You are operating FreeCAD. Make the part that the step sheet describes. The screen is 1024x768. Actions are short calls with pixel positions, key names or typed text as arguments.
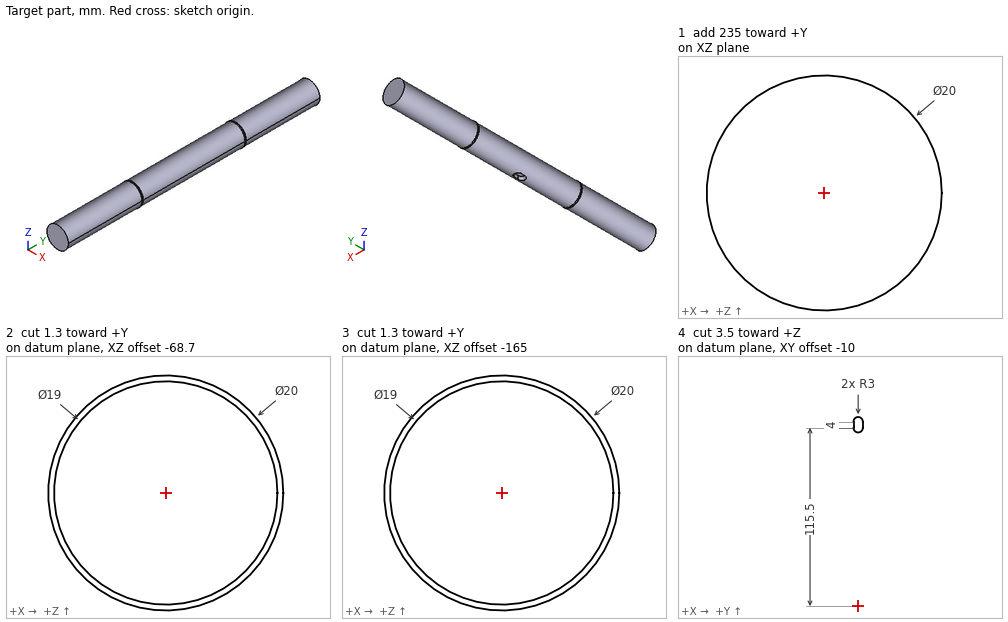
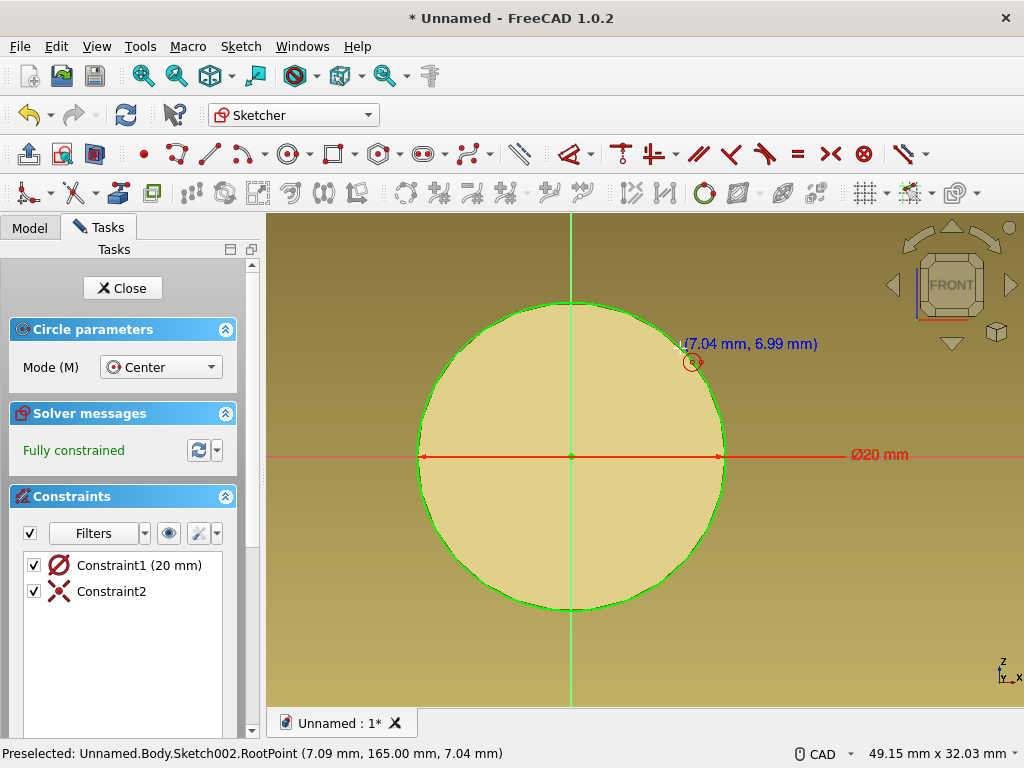
click(571, 457)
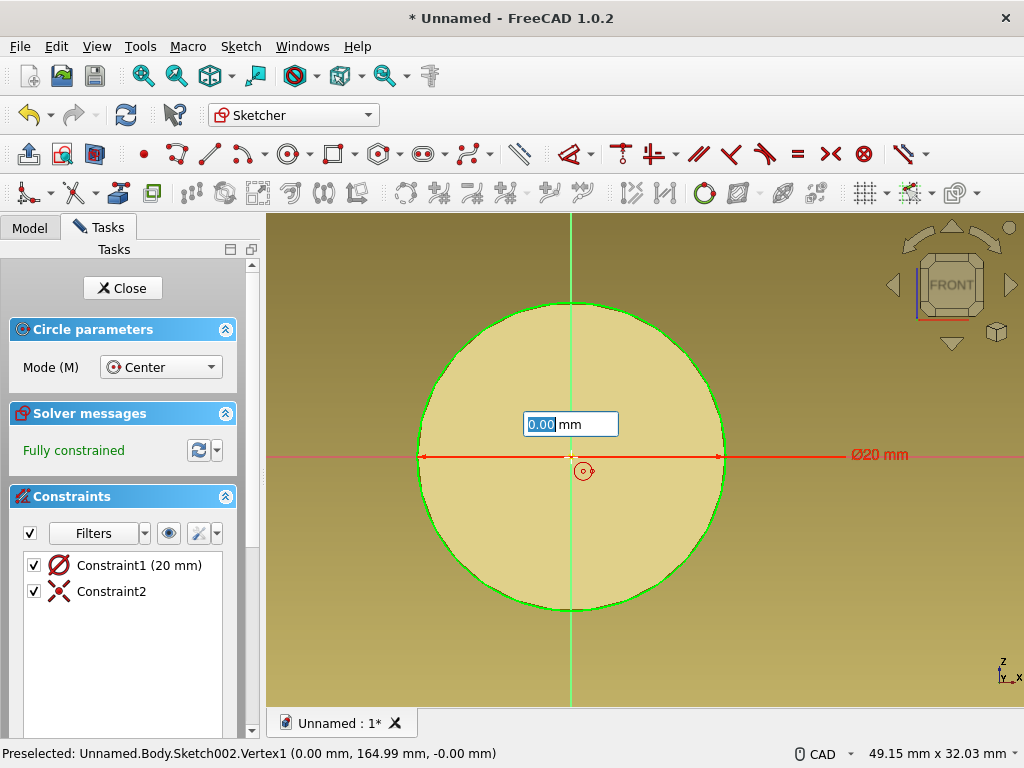
scroll(675, 353, up, 4)
move(674, 353)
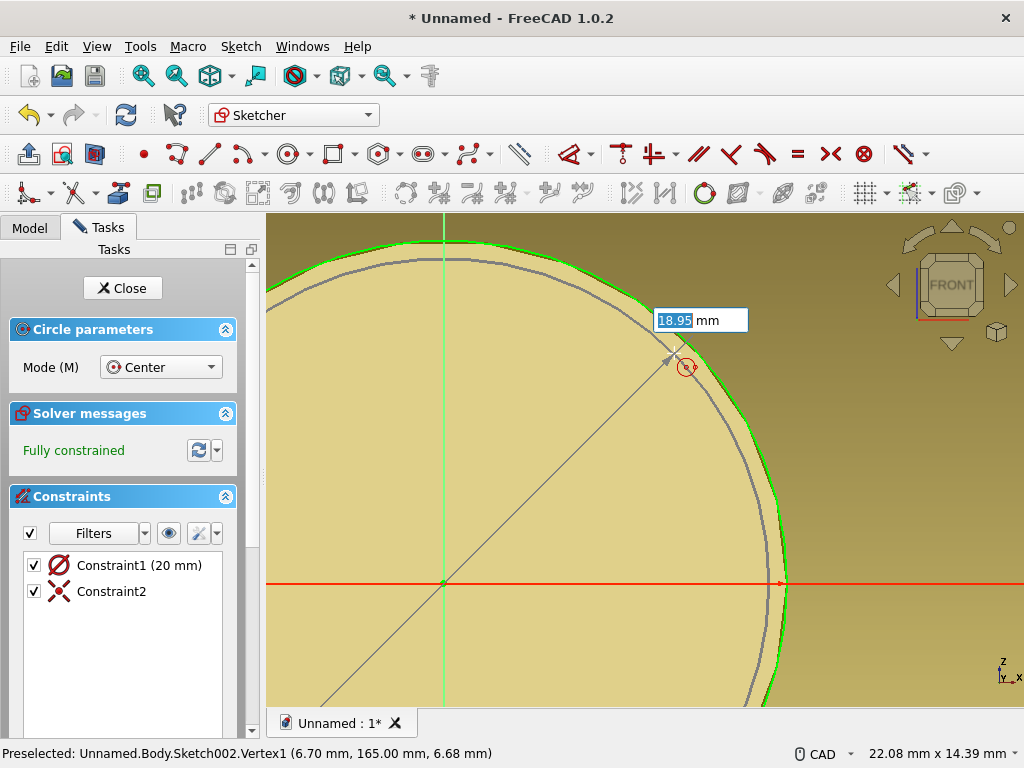
text(19)
key(Return)
key(Escape)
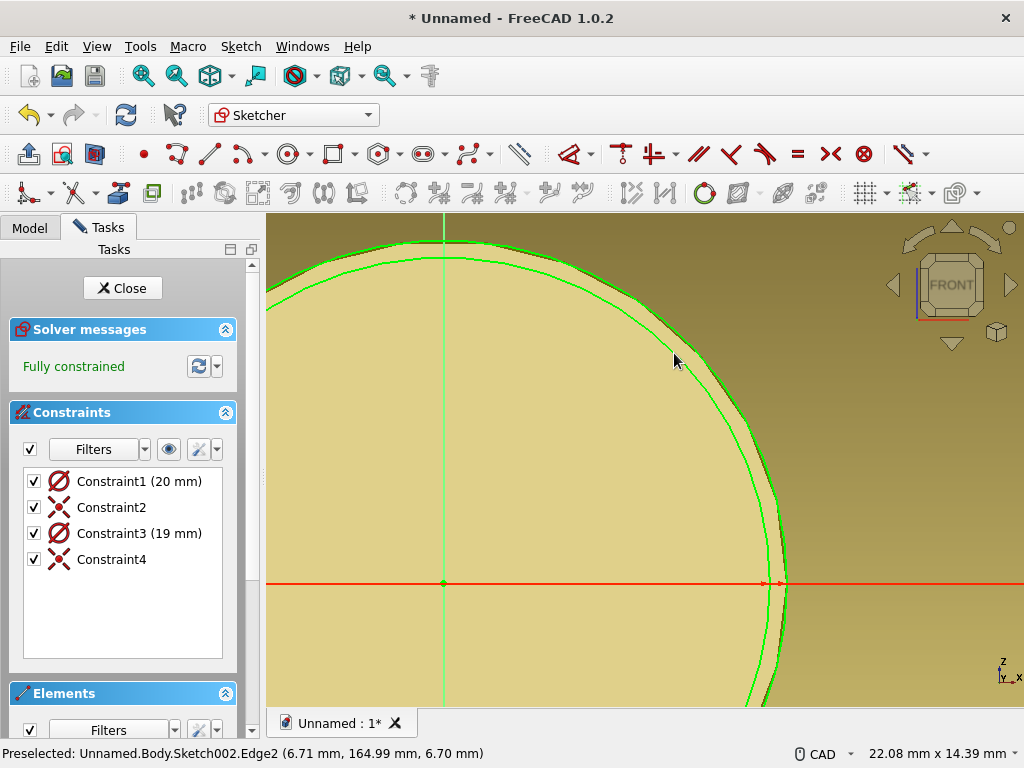
click(123, 288)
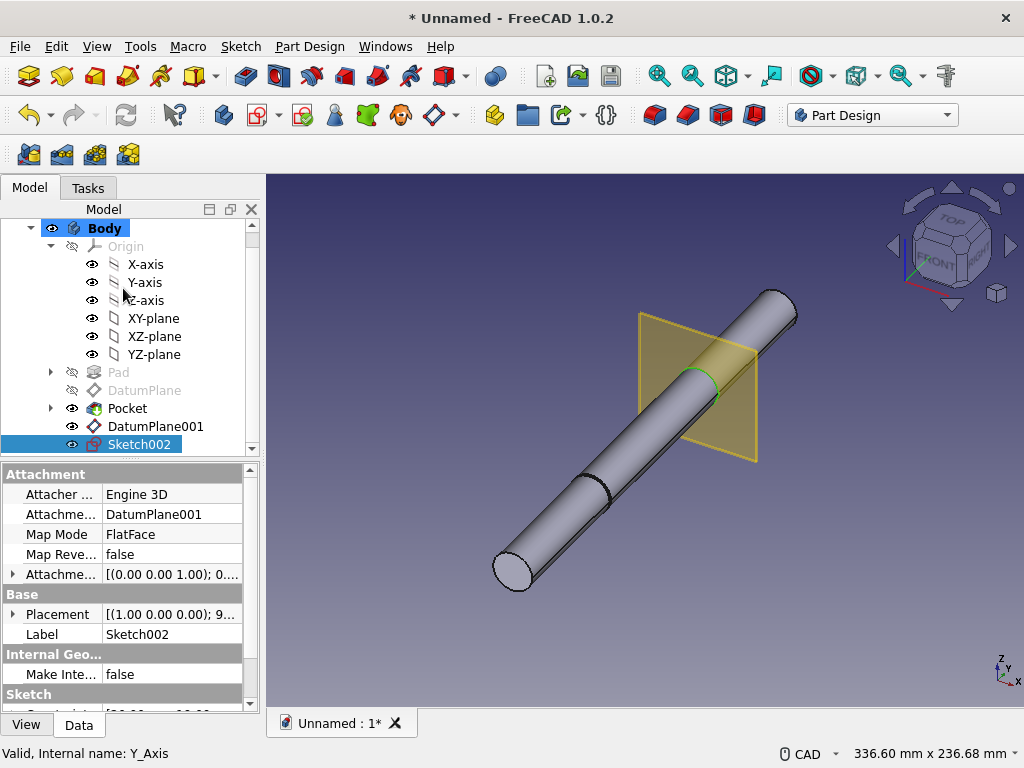
click(246, 76)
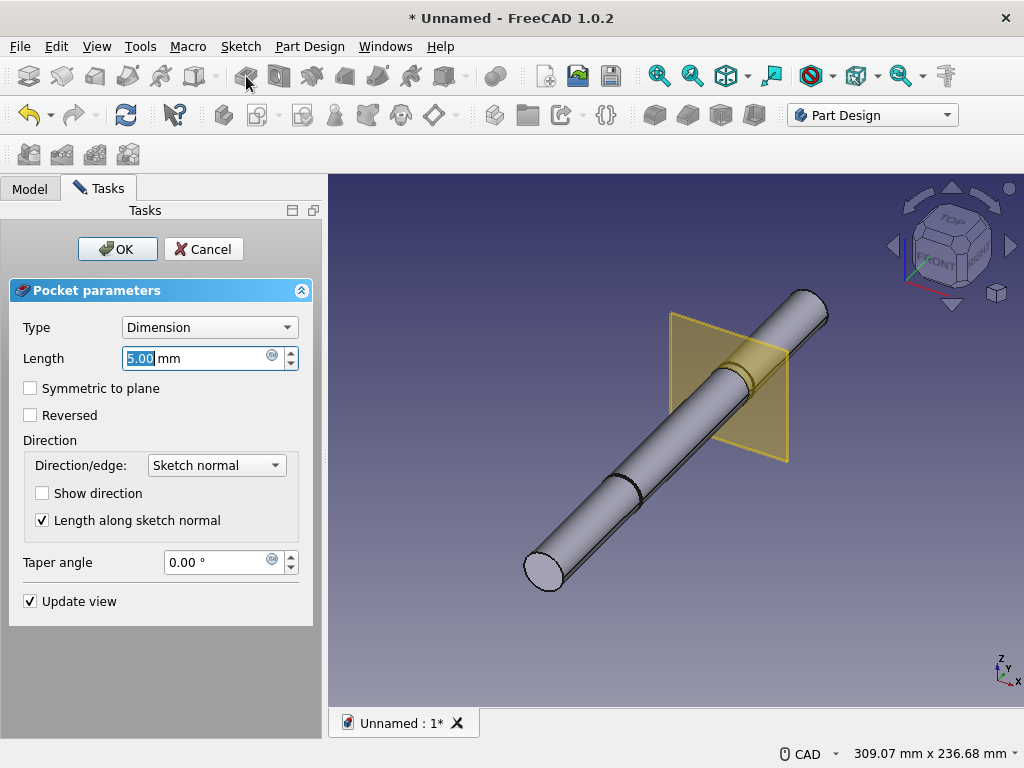
text(1.3)
key(Tab)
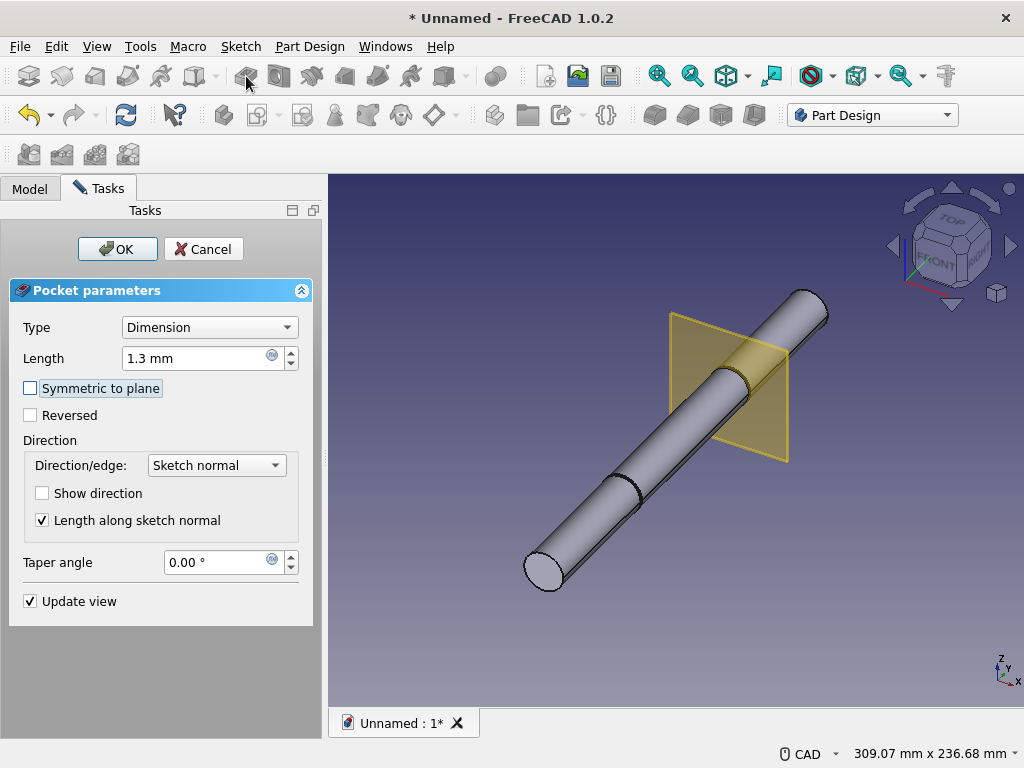
click(118, 249)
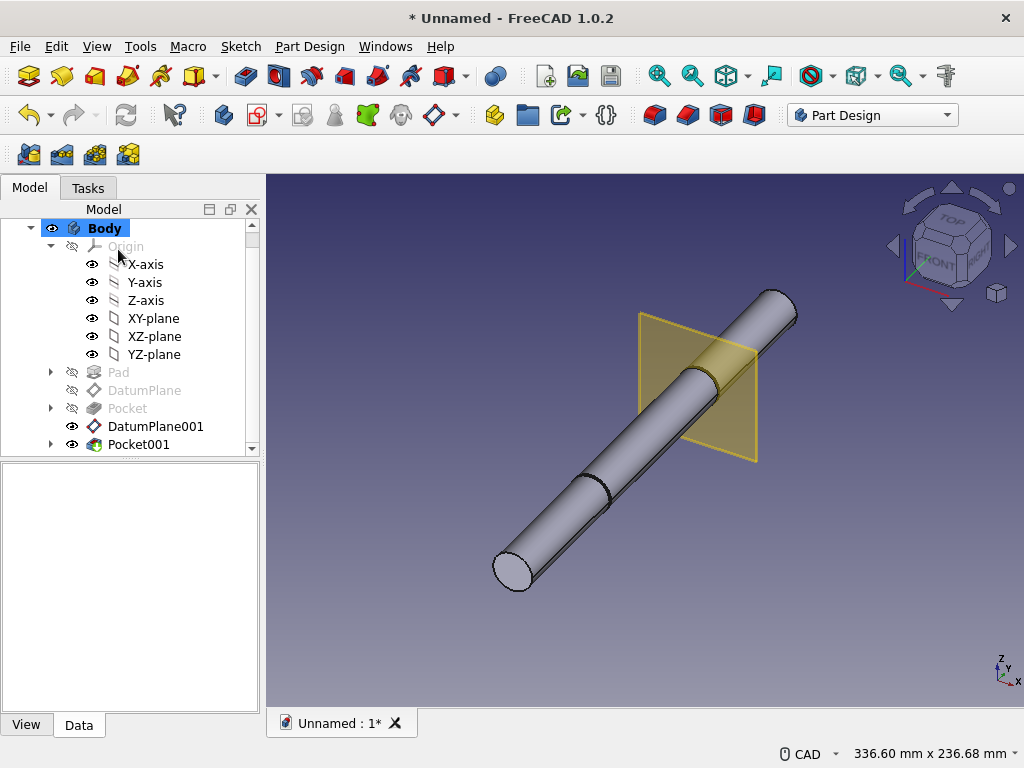
click(117, 426)
key(space)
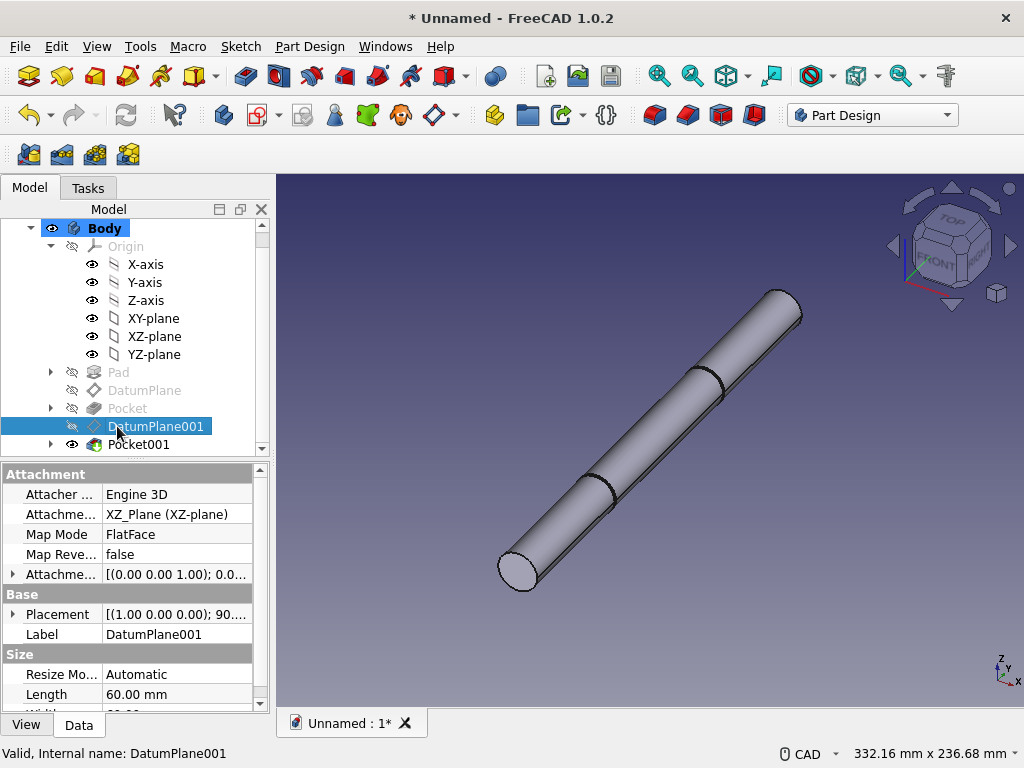
click(137, 318)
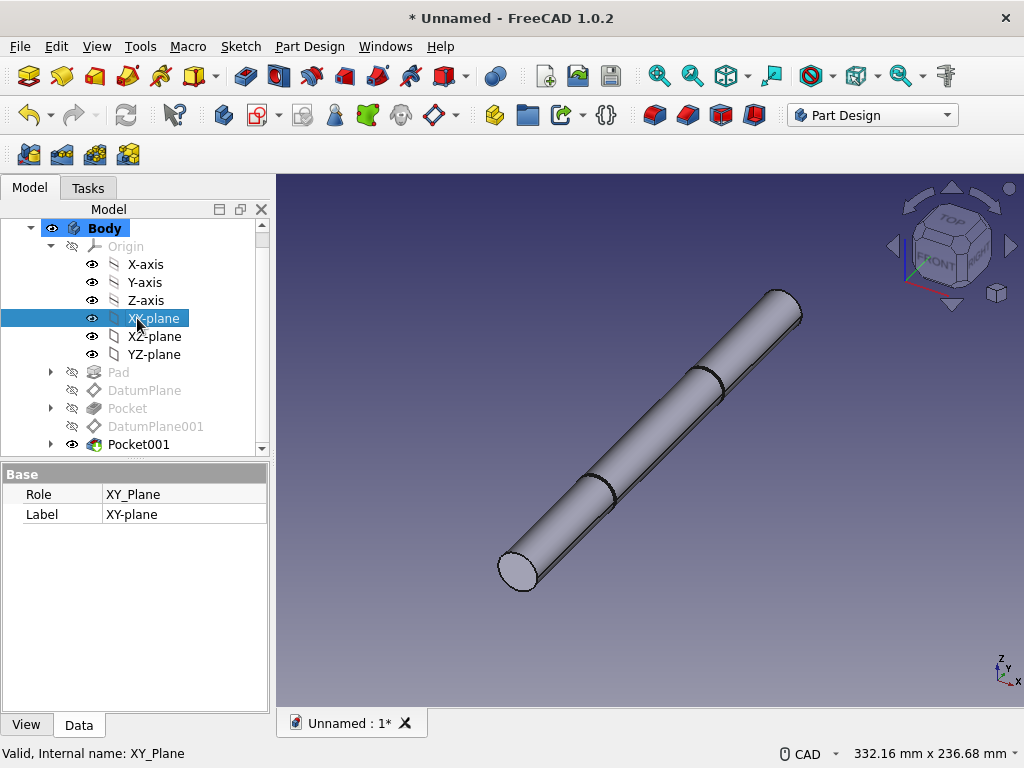
click(434, 116)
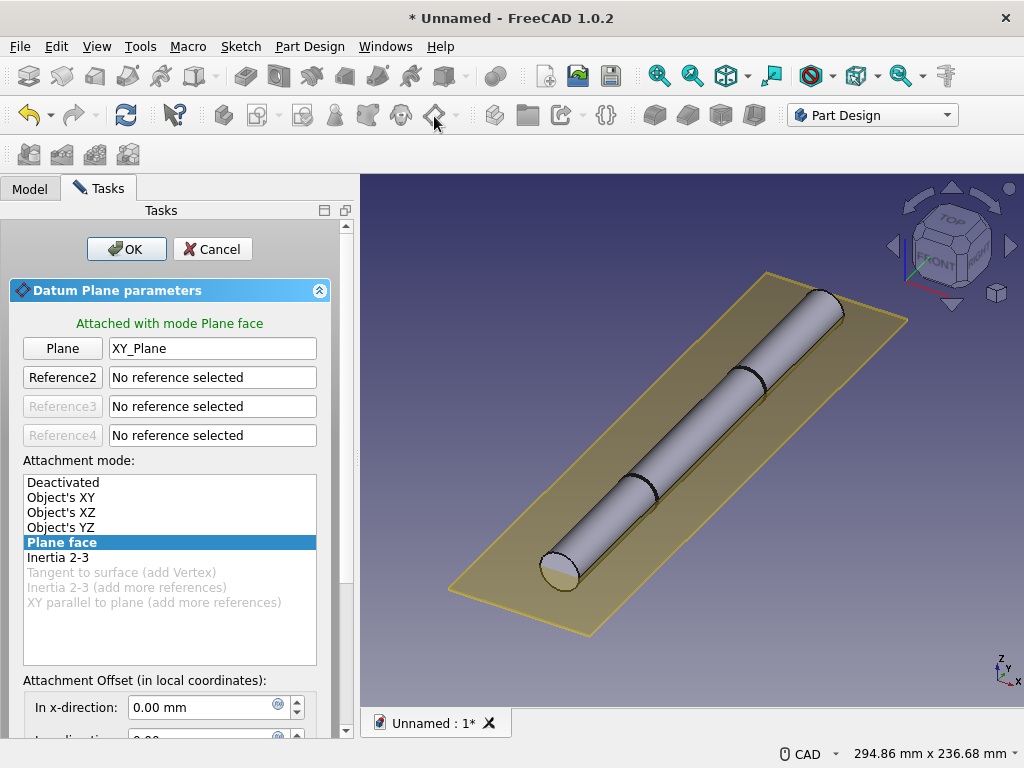
scroll(346, 479, down, 2)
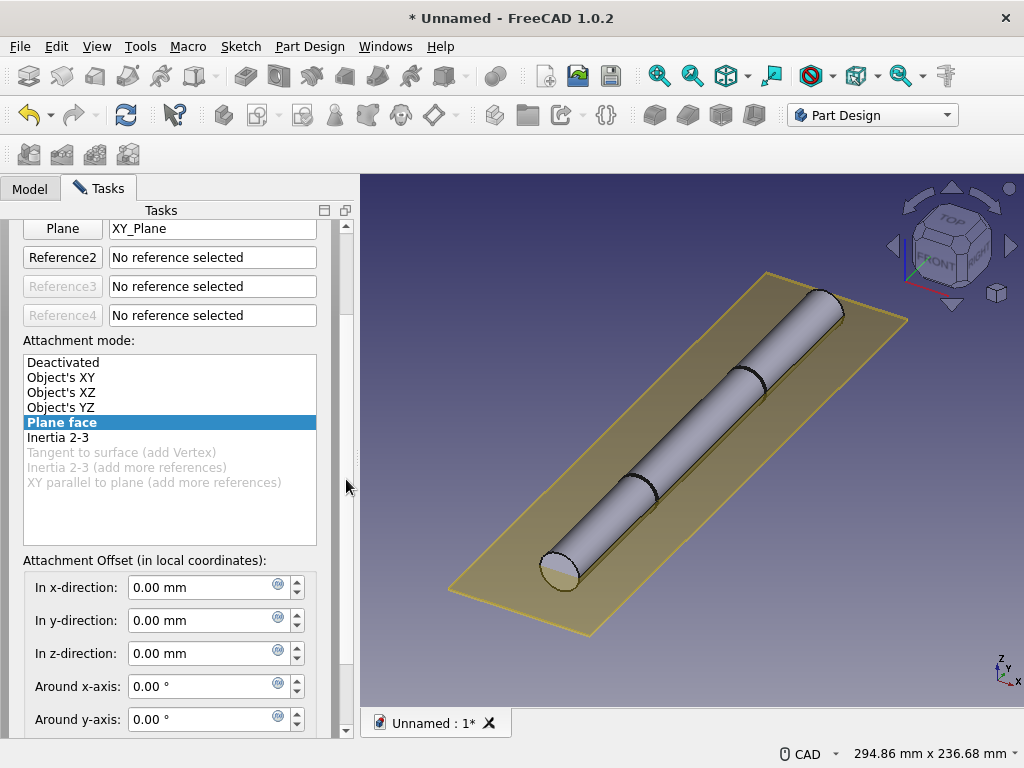
triple_click(210, 654)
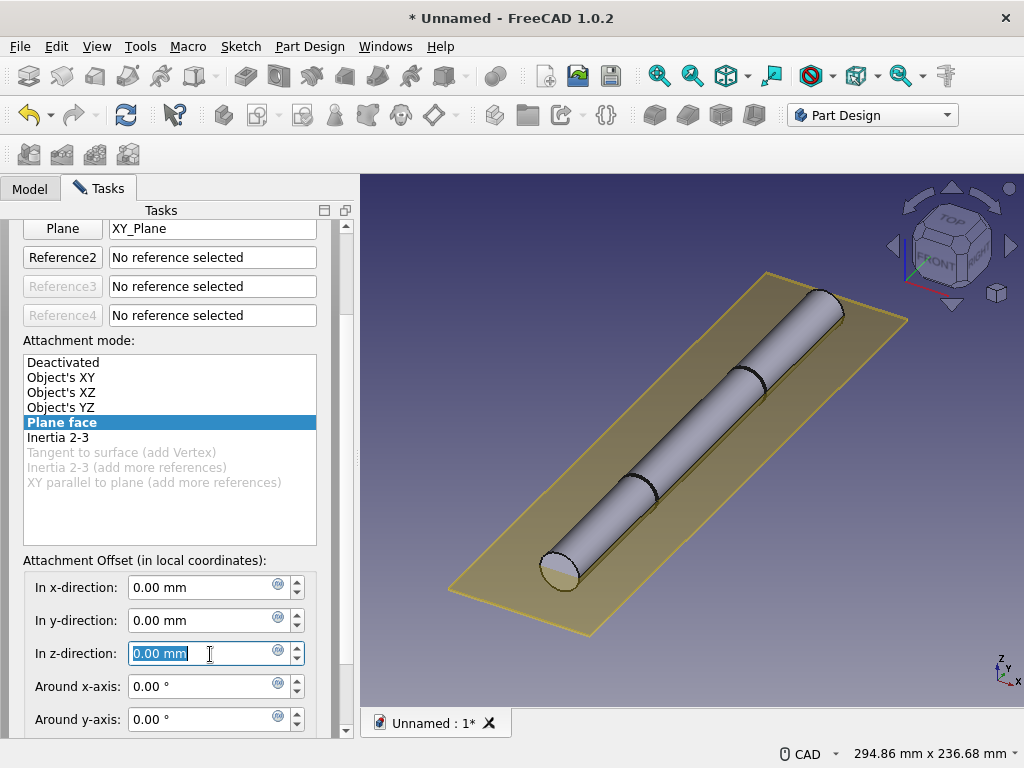
text(-10)
key(Tab)